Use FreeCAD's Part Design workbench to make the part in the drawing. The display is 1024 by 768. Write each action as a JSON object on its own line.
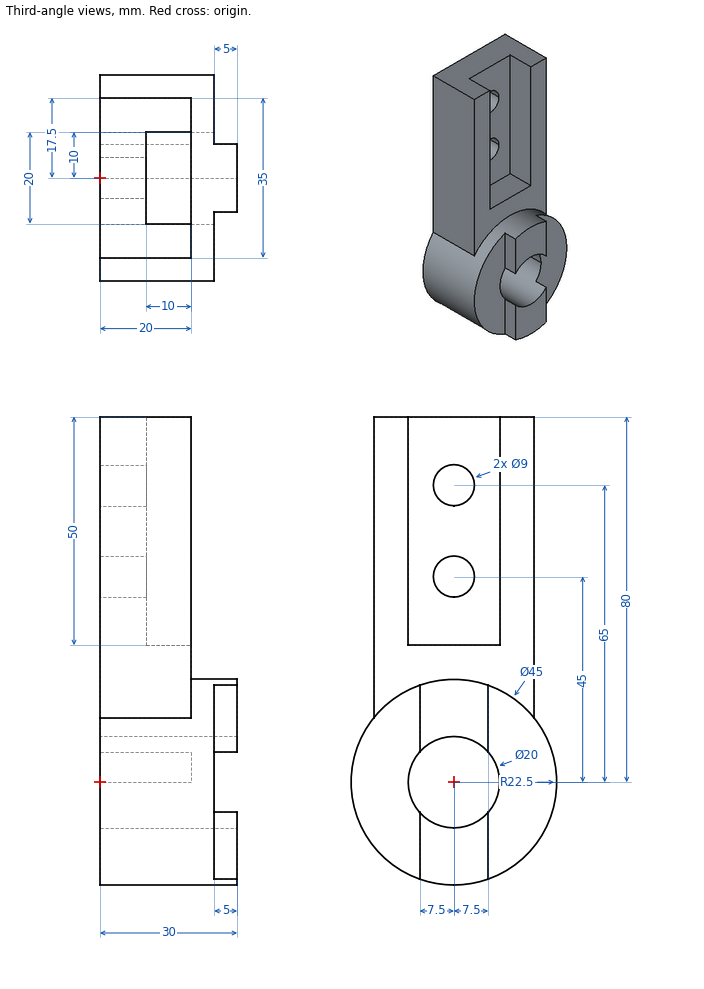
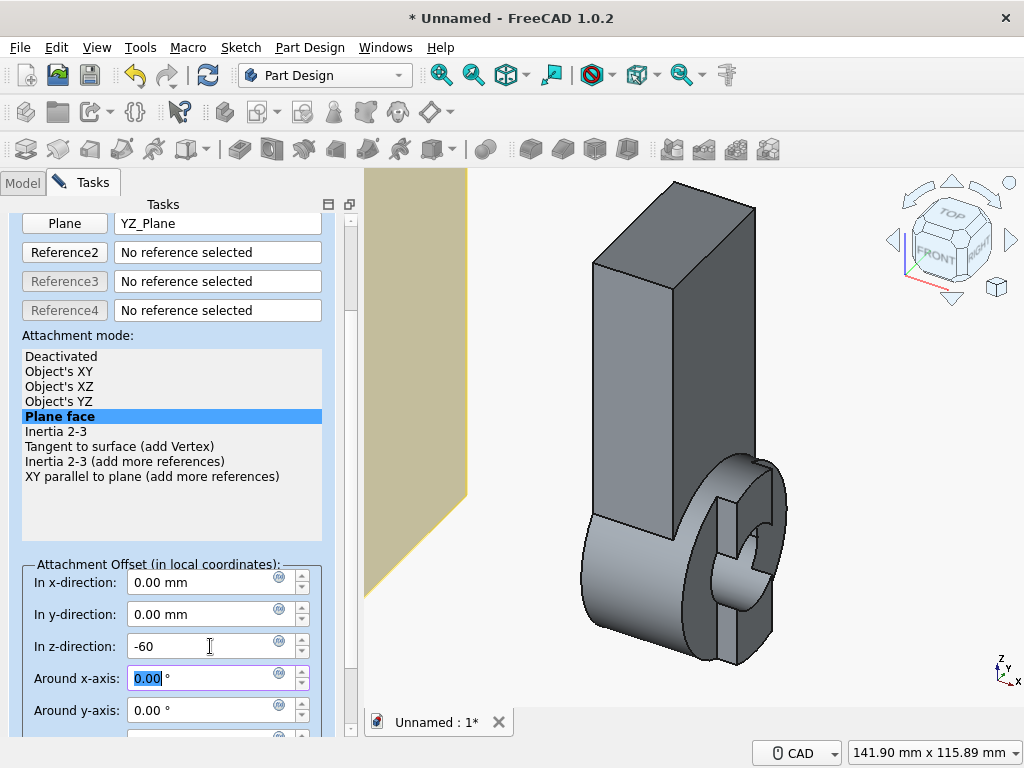
{"action": "scroll", "coordinate": [351, 475], "scroll_direction": "up", "scroll_amount": 3}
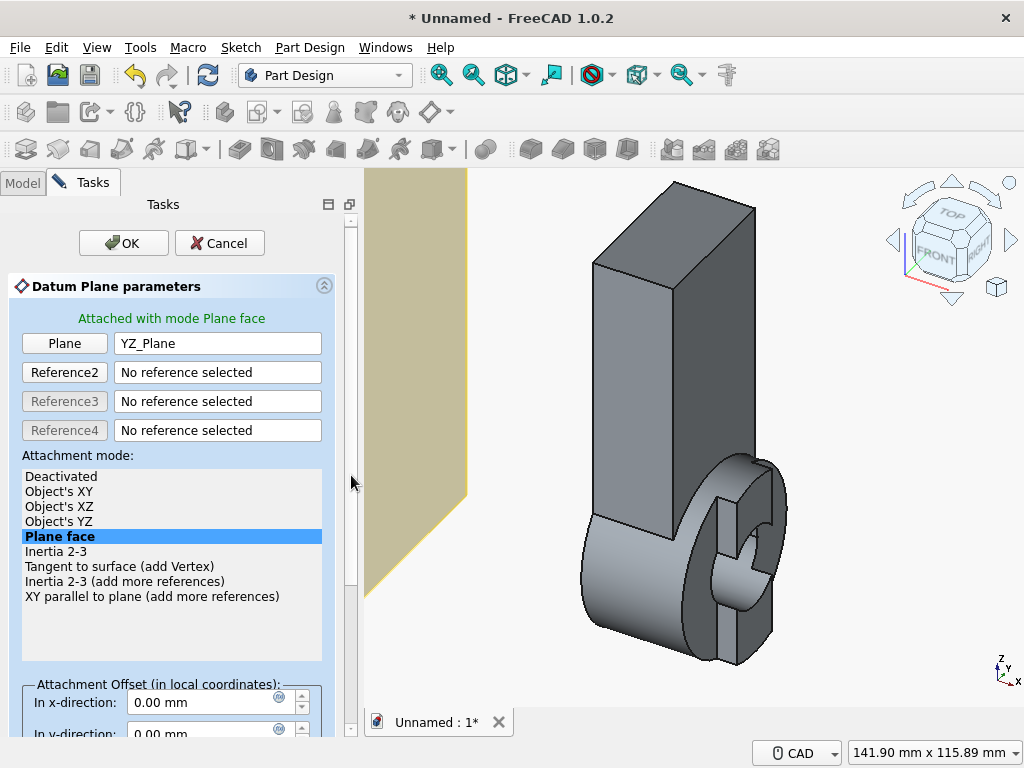
{"action": "left_click", "coordinate": [124, 243]}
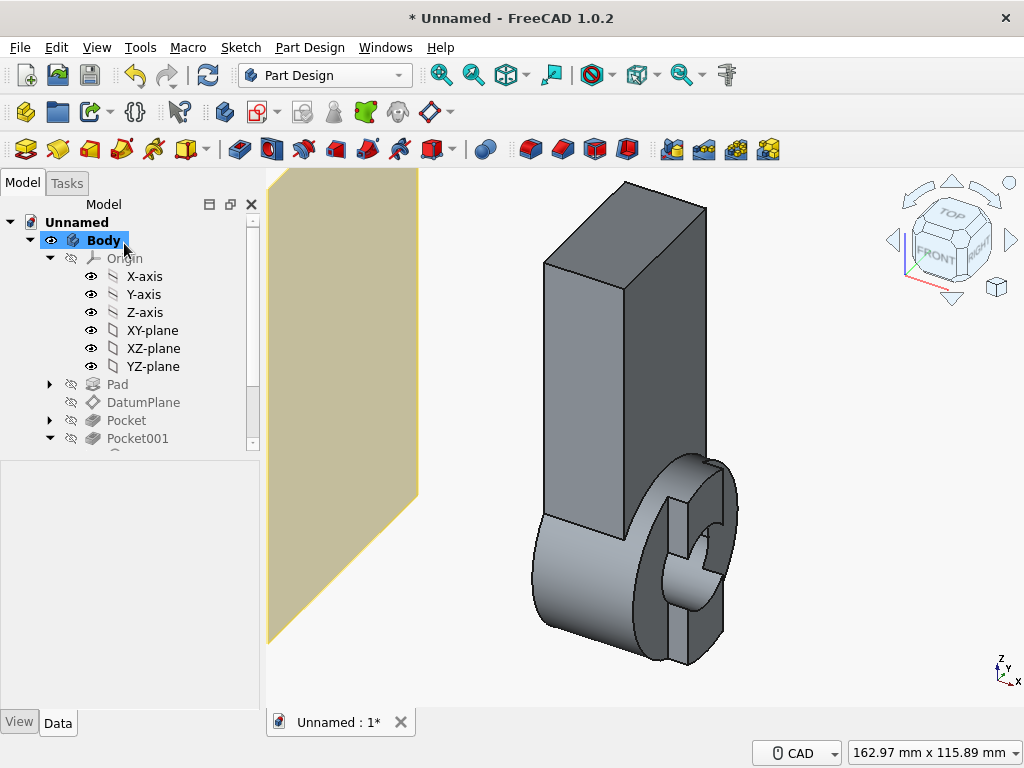
{"action": "scroll", "coordinate": [100, 326], "scroll_direction": "down", "scroll_amount": 3}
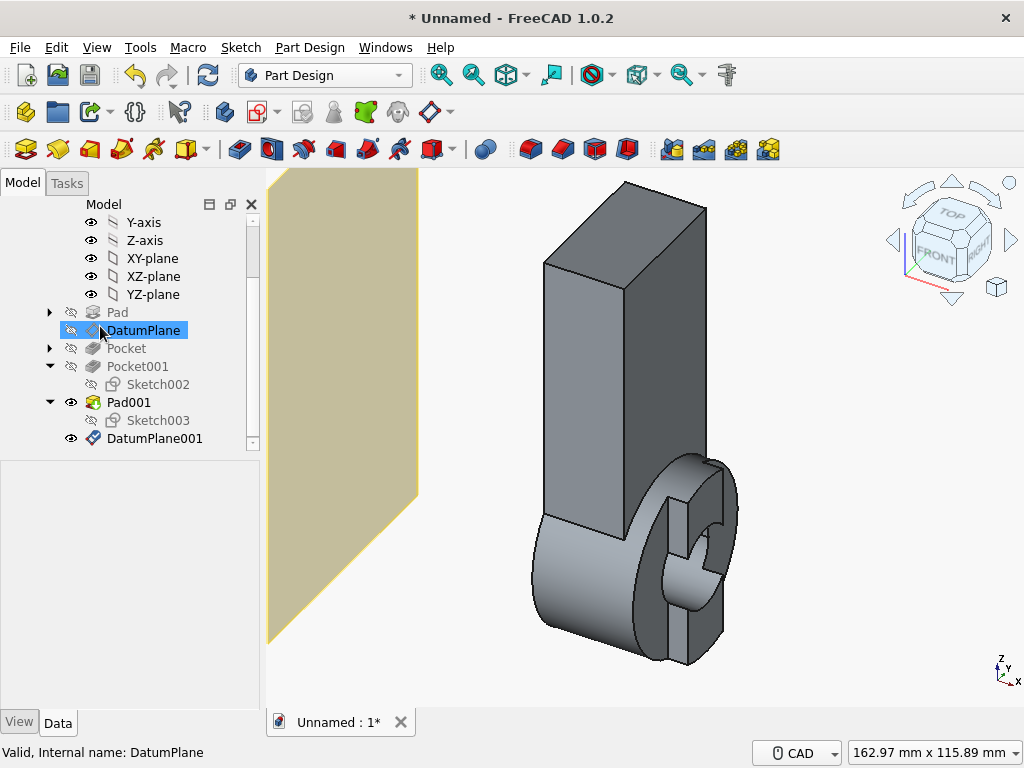
{"action": "left_click", "coordinate": [116, 438]}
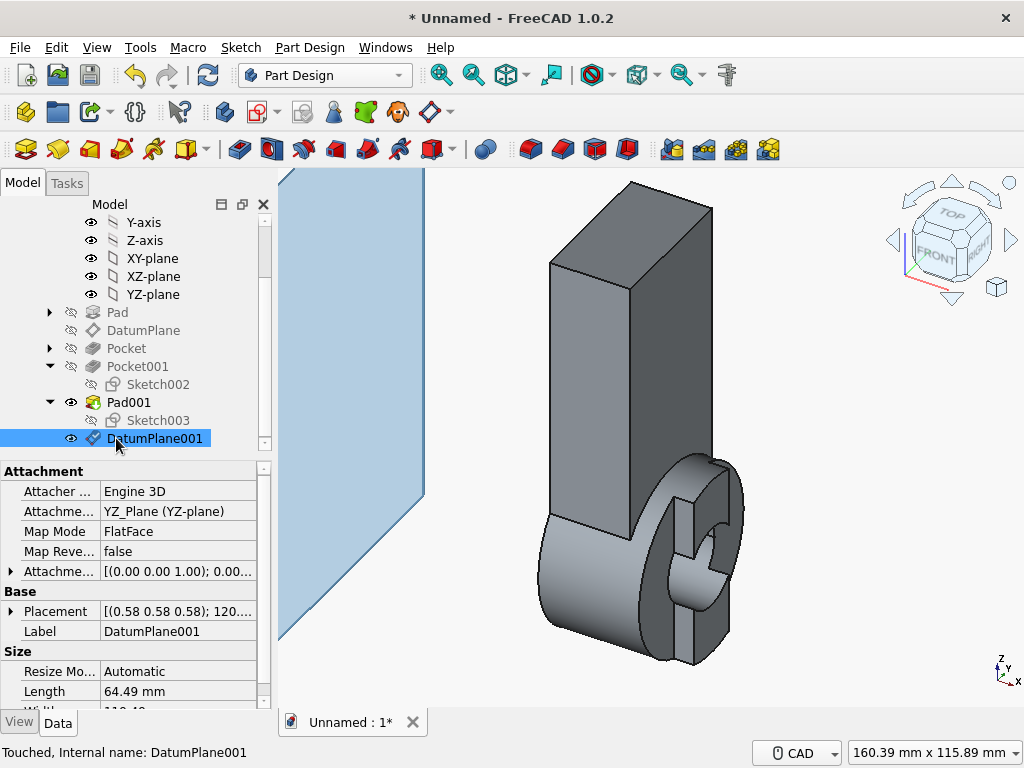
{"action": "left_click", "coordinate": [258, 112]}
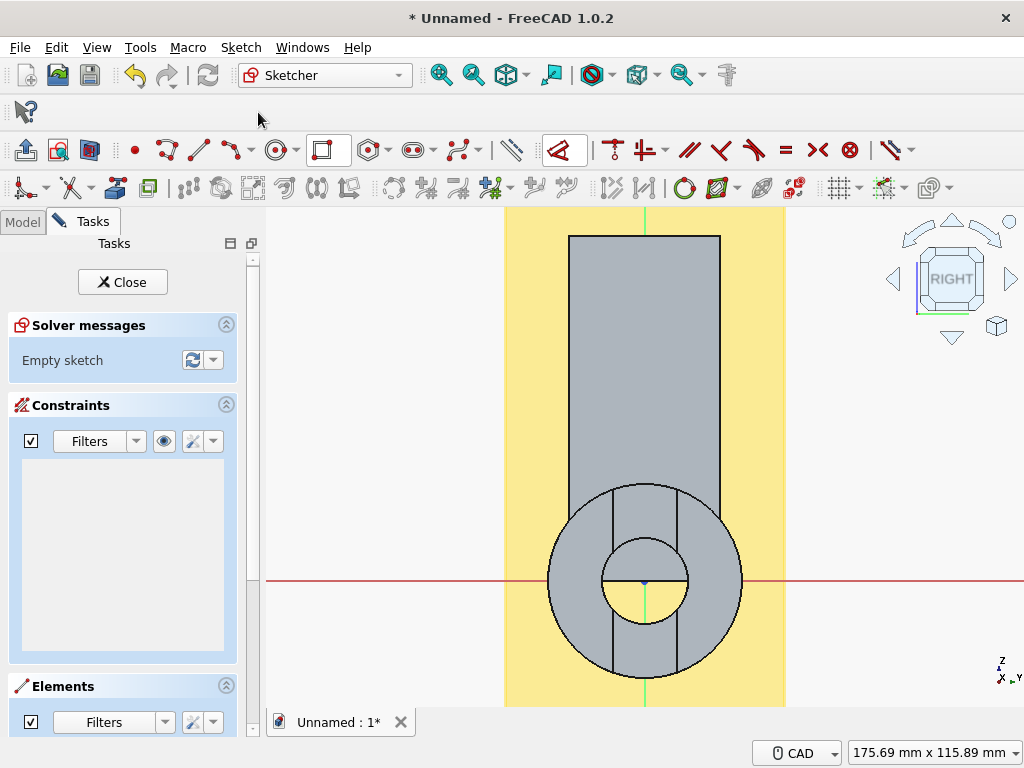
{"action": "left_click", "coordinate": [90, 150]}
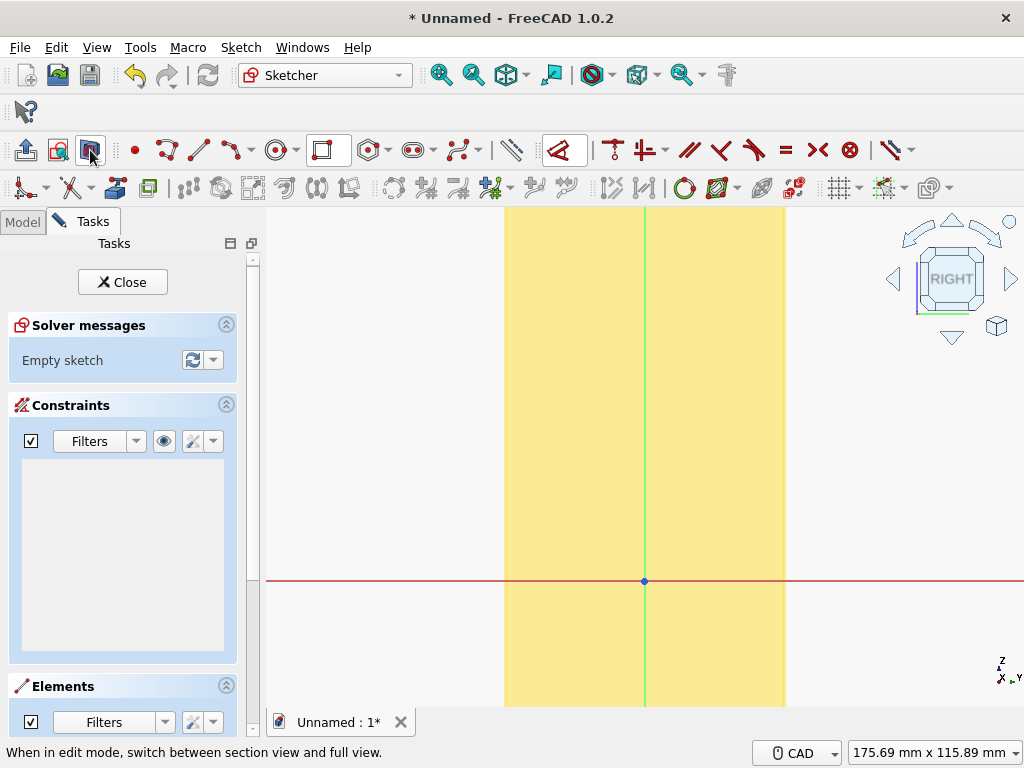
{"action": "scroll", "coordinate": [674, 635], "scroll_direction": "up", "scroll_amount": 6}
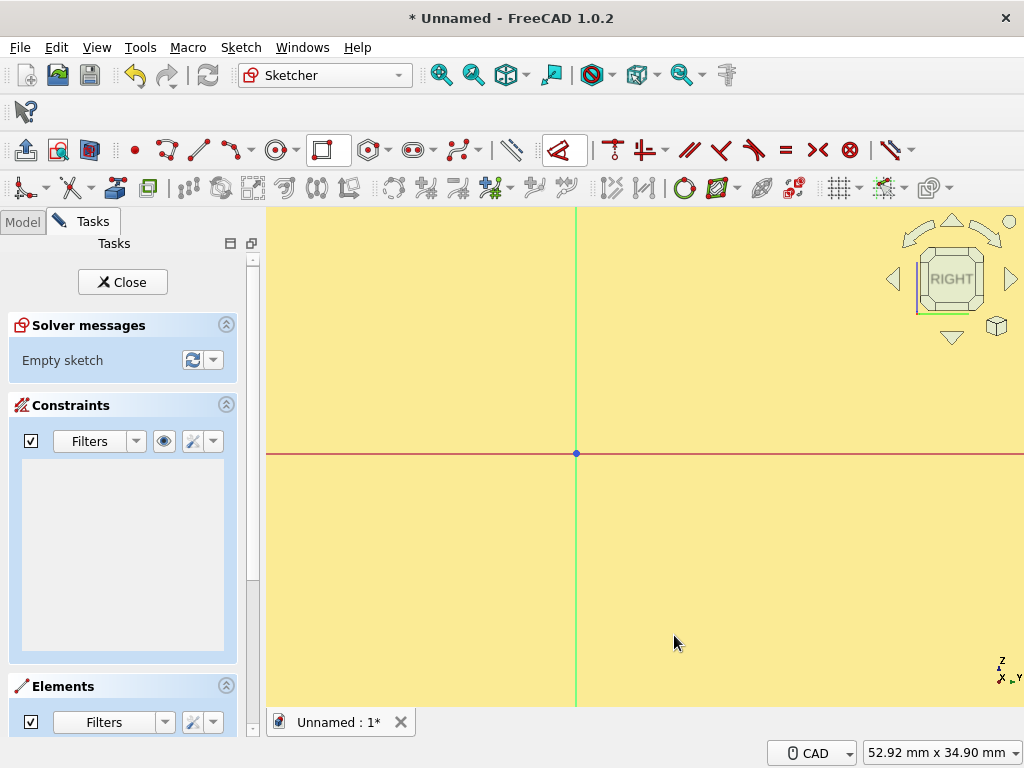
{"action": "left_click", "coordinate": [276, 150]}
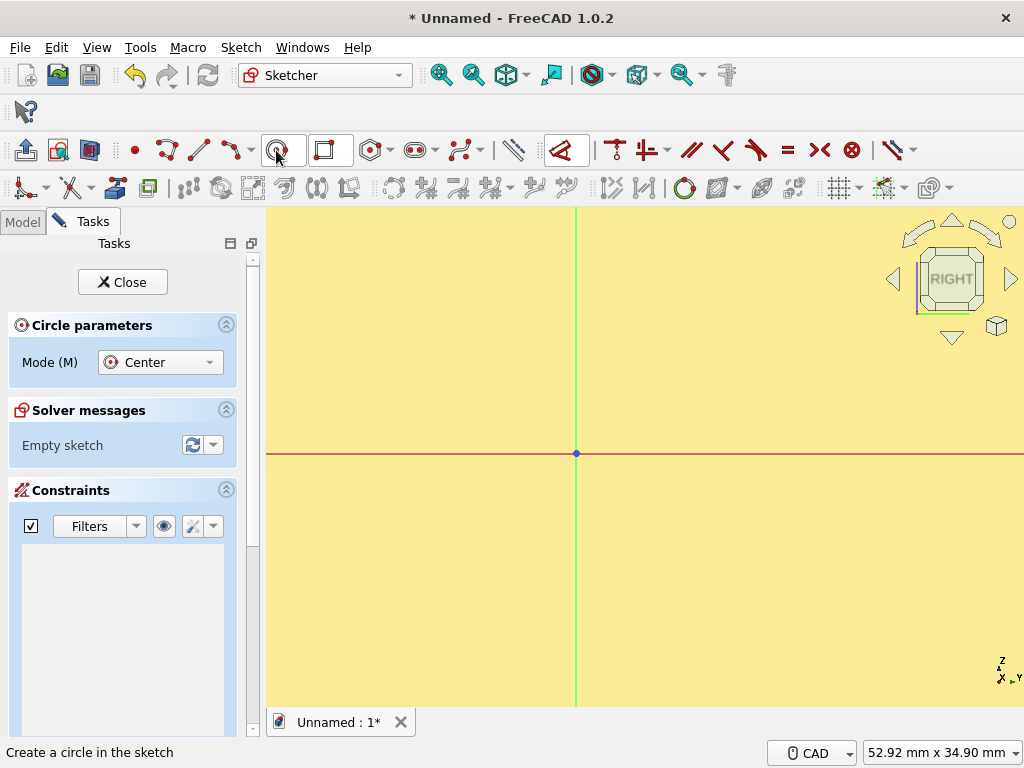
{"action": "left_click", "coordinate": [576, 454]}
{"action": "mouse_move", "coordinate": [678, 353]}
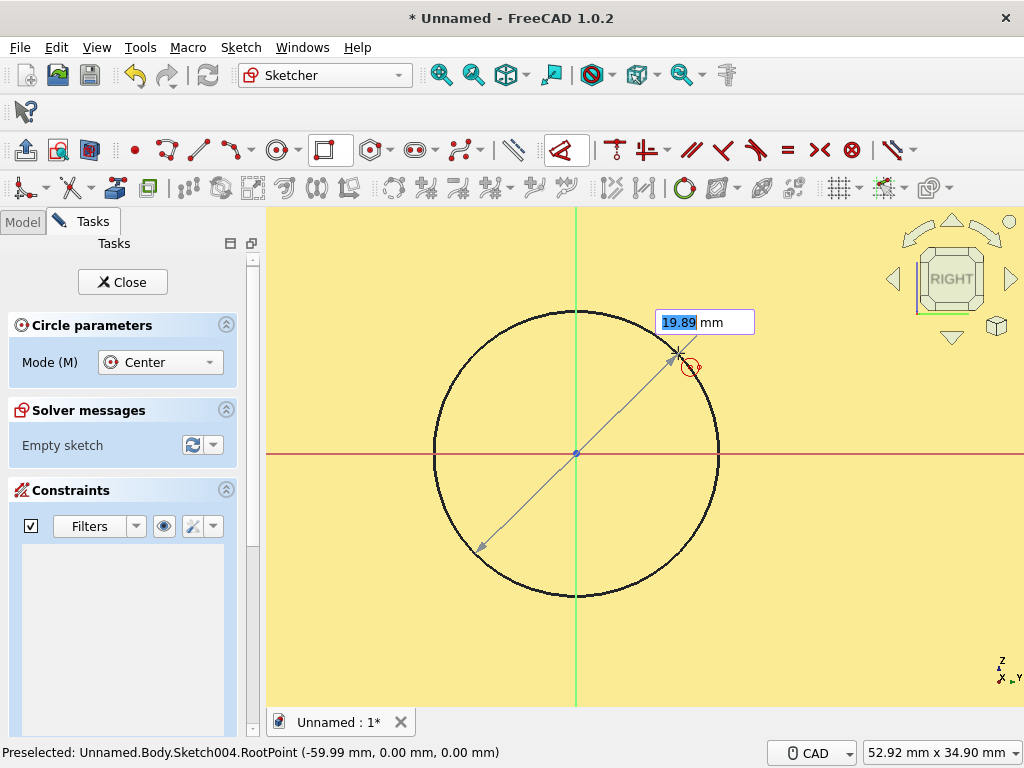
{"action": "type", "text": "20"}
{"action": "key", "text": "Return"}
{"action": "key", "text": "Escape"}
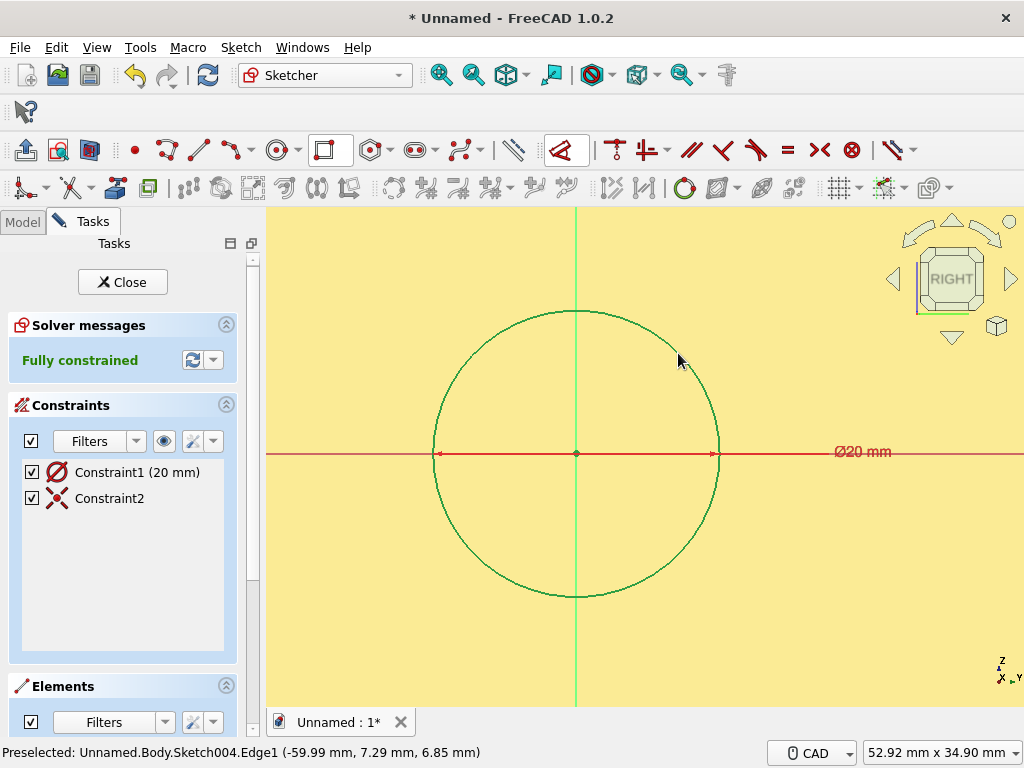
{"action": "left_click", "coordinate": [123, 282]}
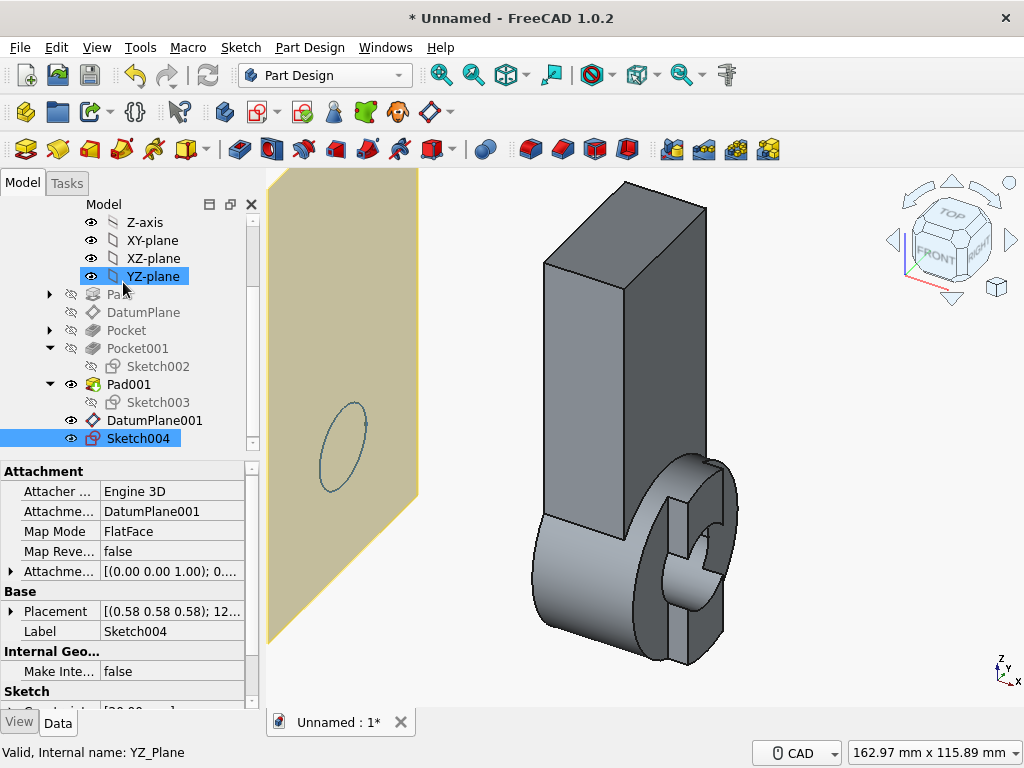
{"action": "left_click", "coordinate": [240, 150]}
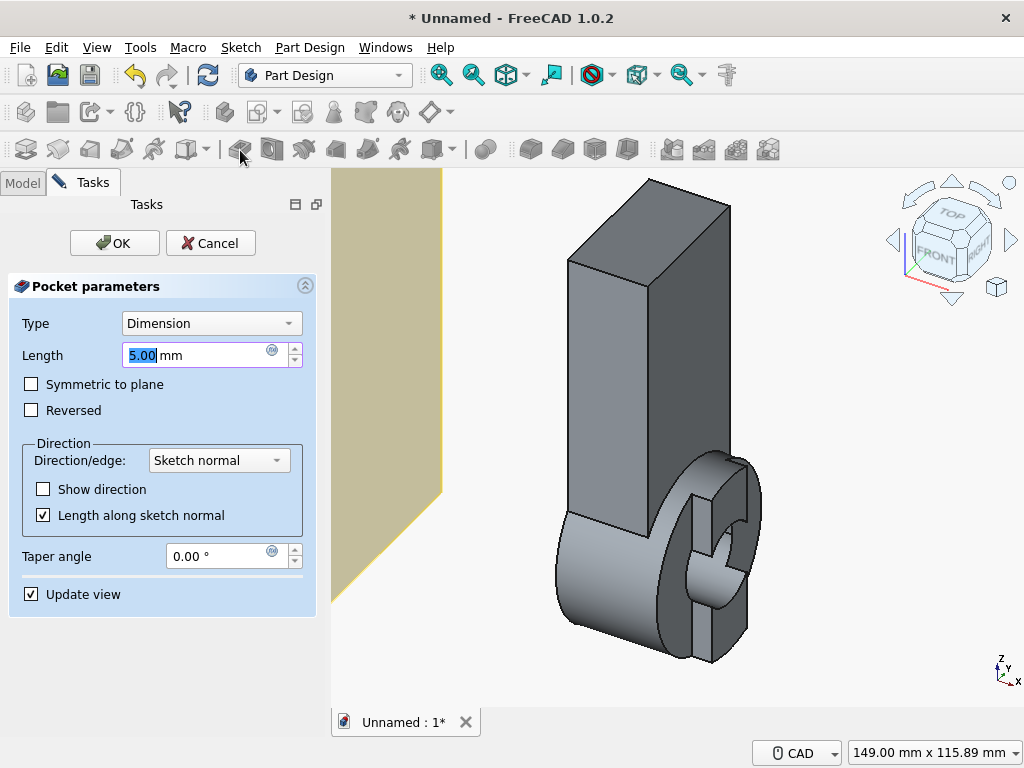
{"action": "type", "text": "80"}
{"action": "key", "text": "Tab"}